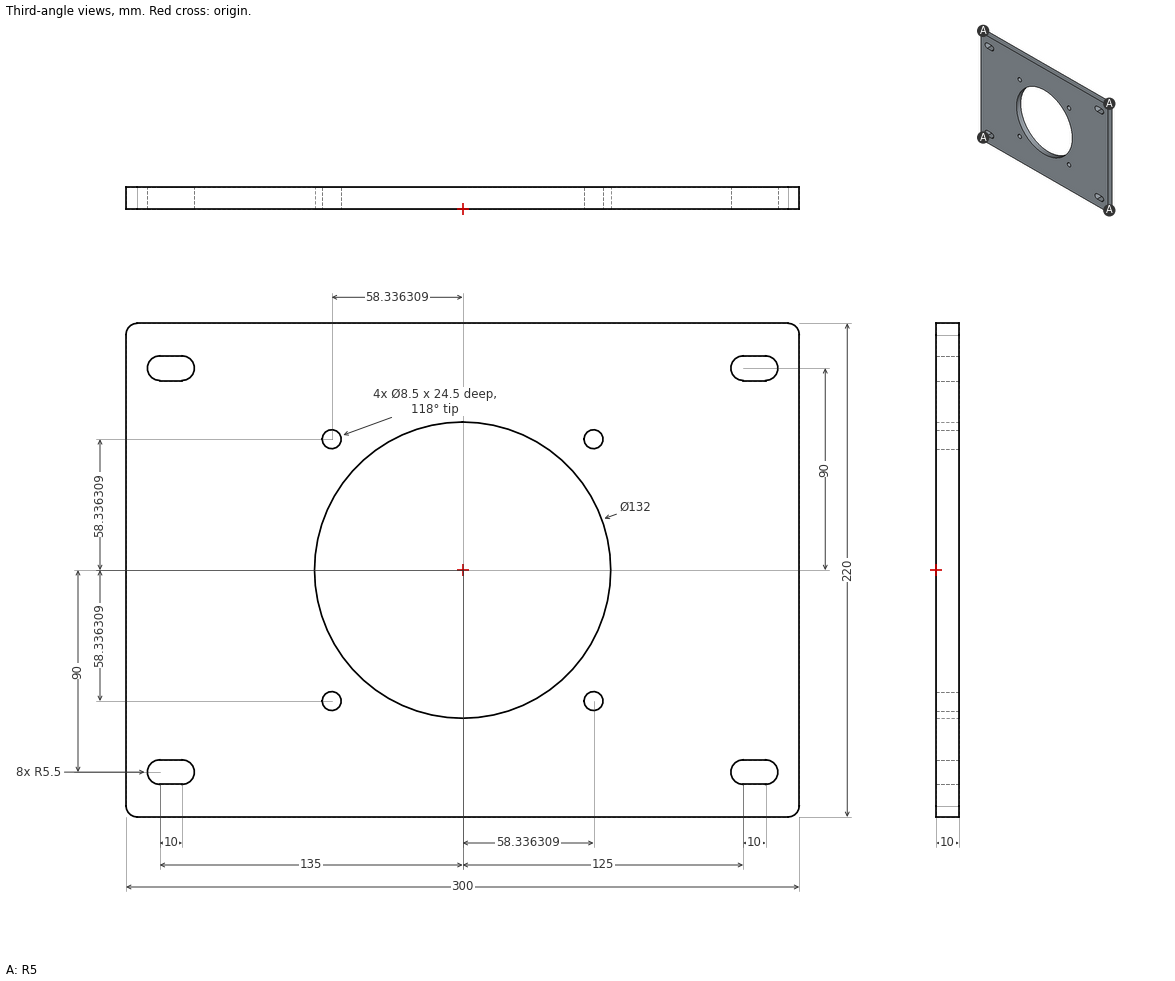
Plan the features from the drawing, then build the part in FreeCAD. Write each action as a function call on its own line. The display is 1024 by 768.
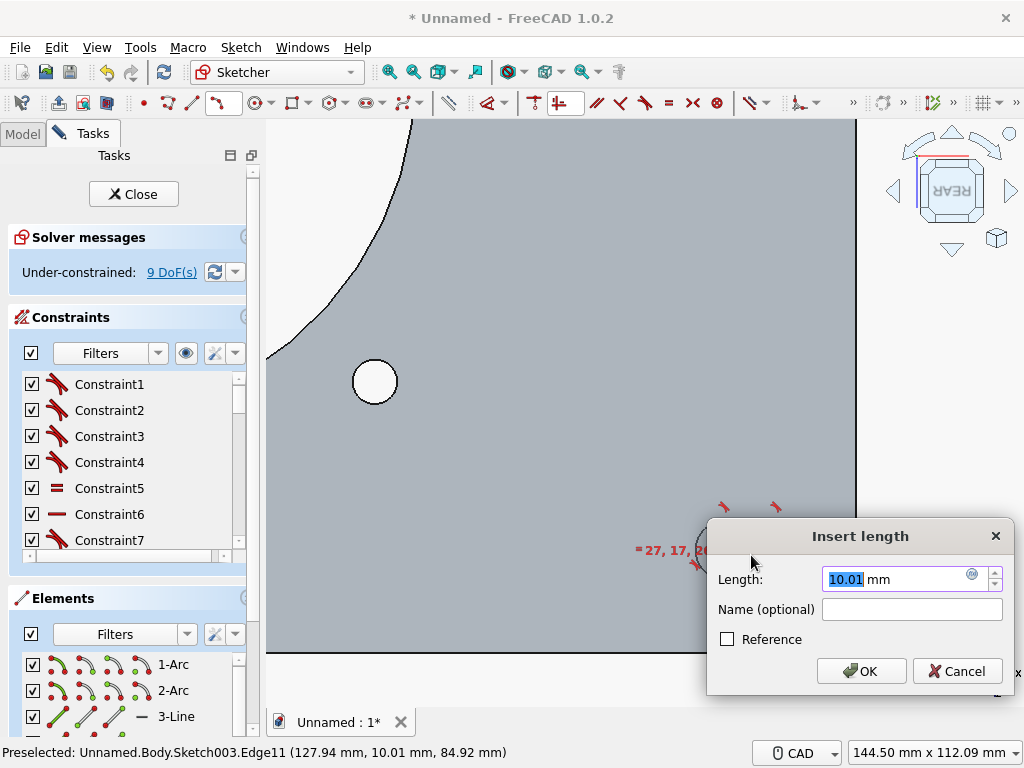
text(10)
key(Return)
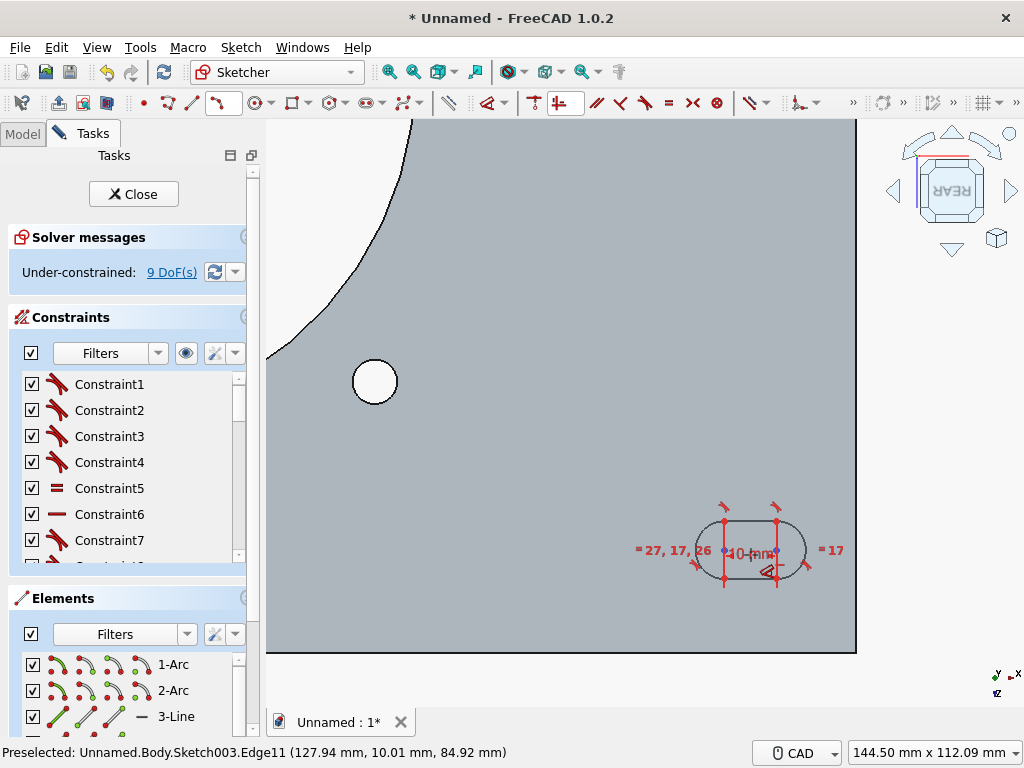
scroll(743, 523, down, 7)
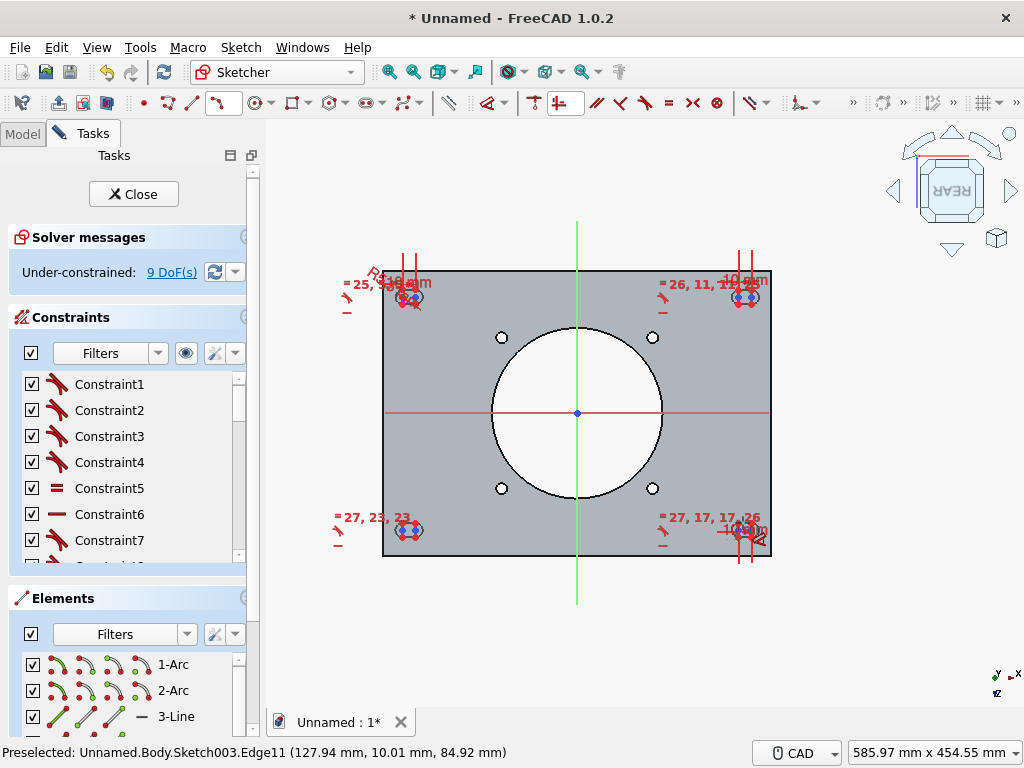
scroll(406, 523, up, 7)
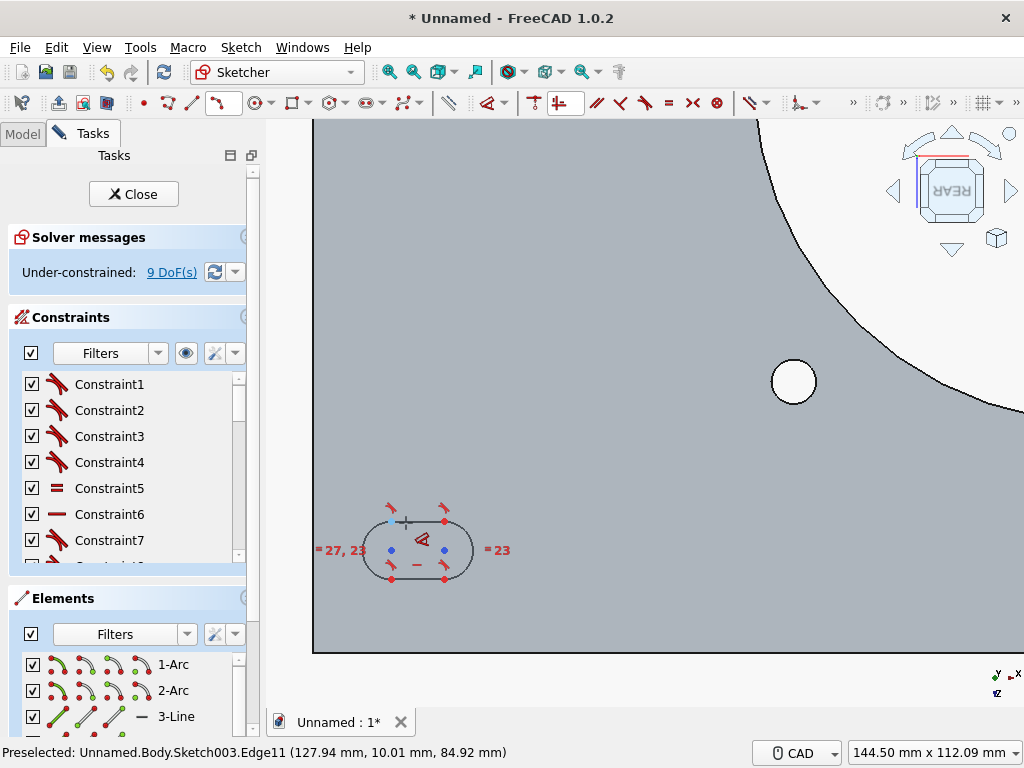
click(407, 522)
click(418, 556)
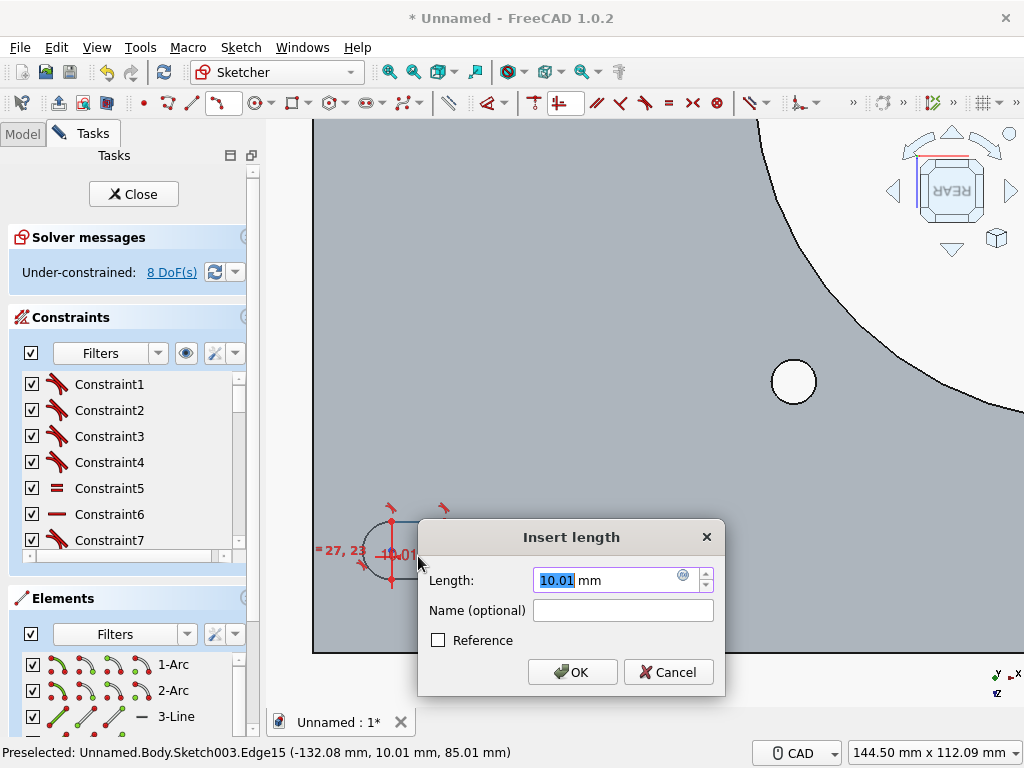
text(10)
key(Return)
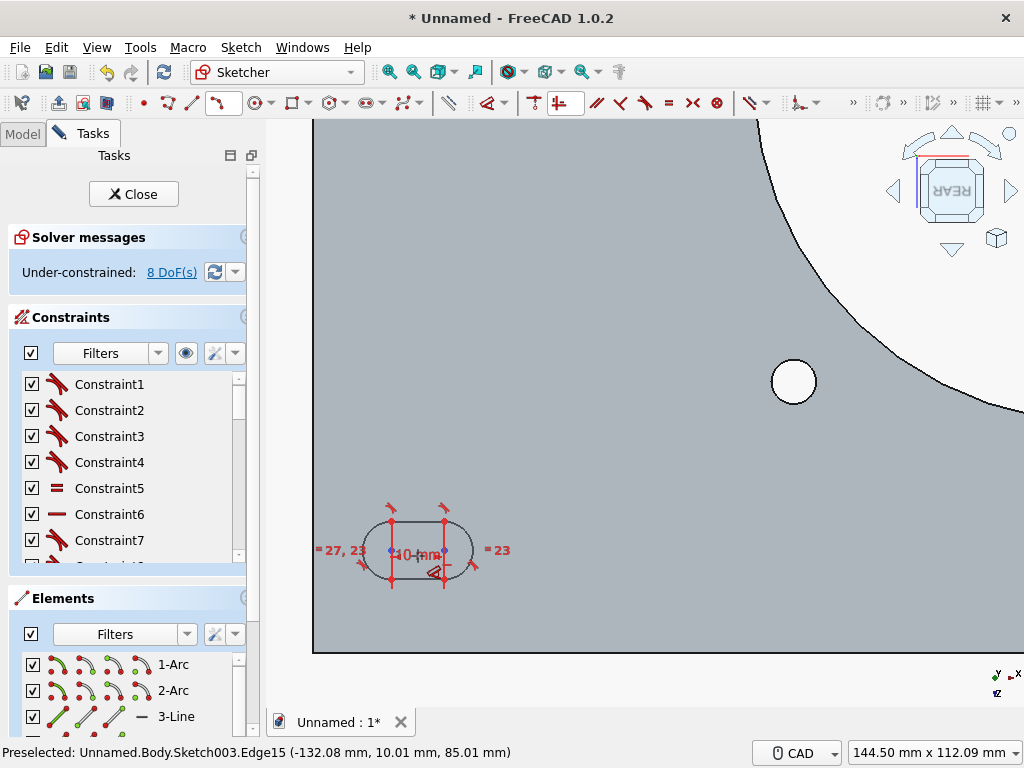
scroll(405, 523, down, 7)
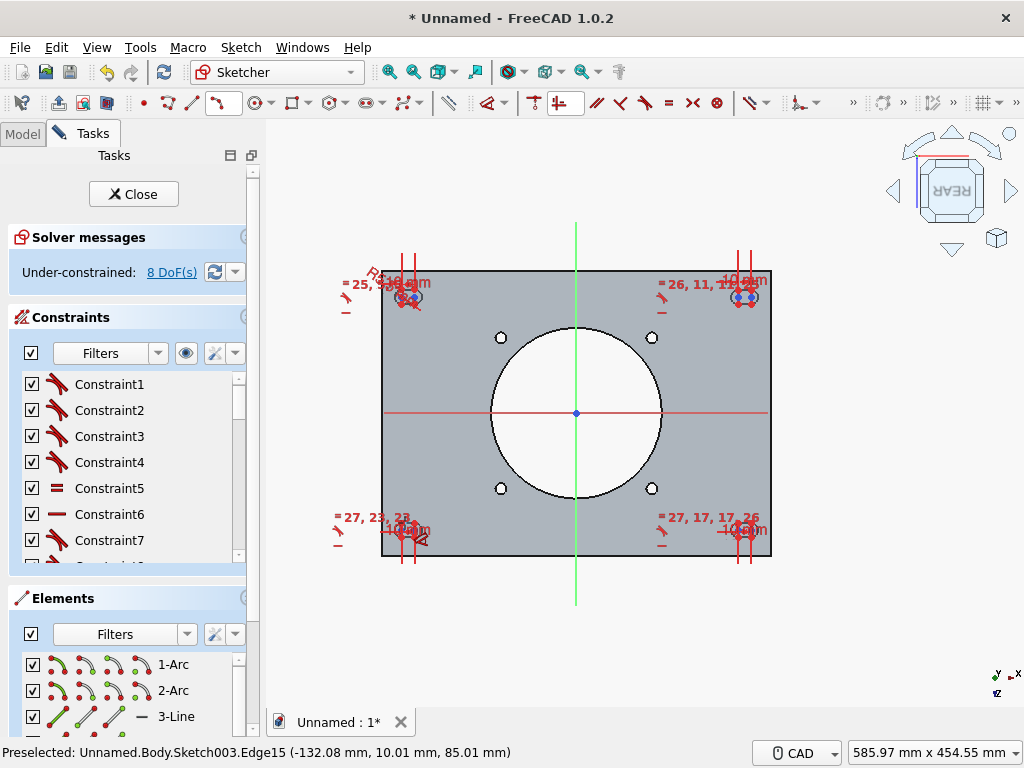
scroll(402, 297, up, 3)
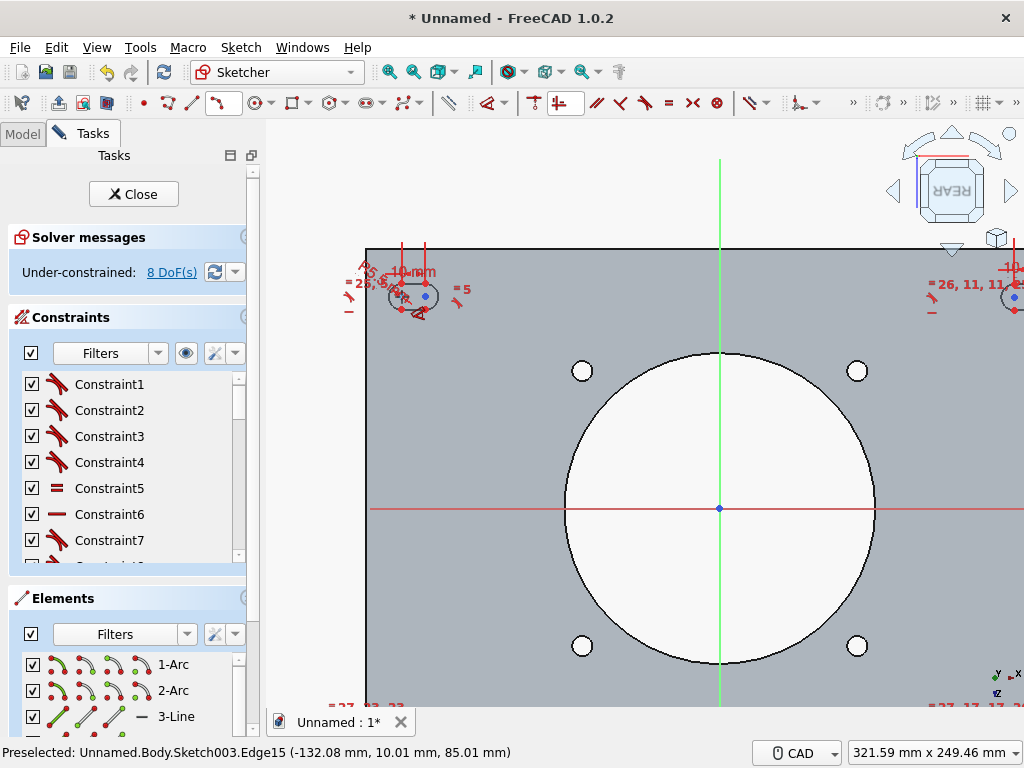
click(402, 297)
click(368, 403)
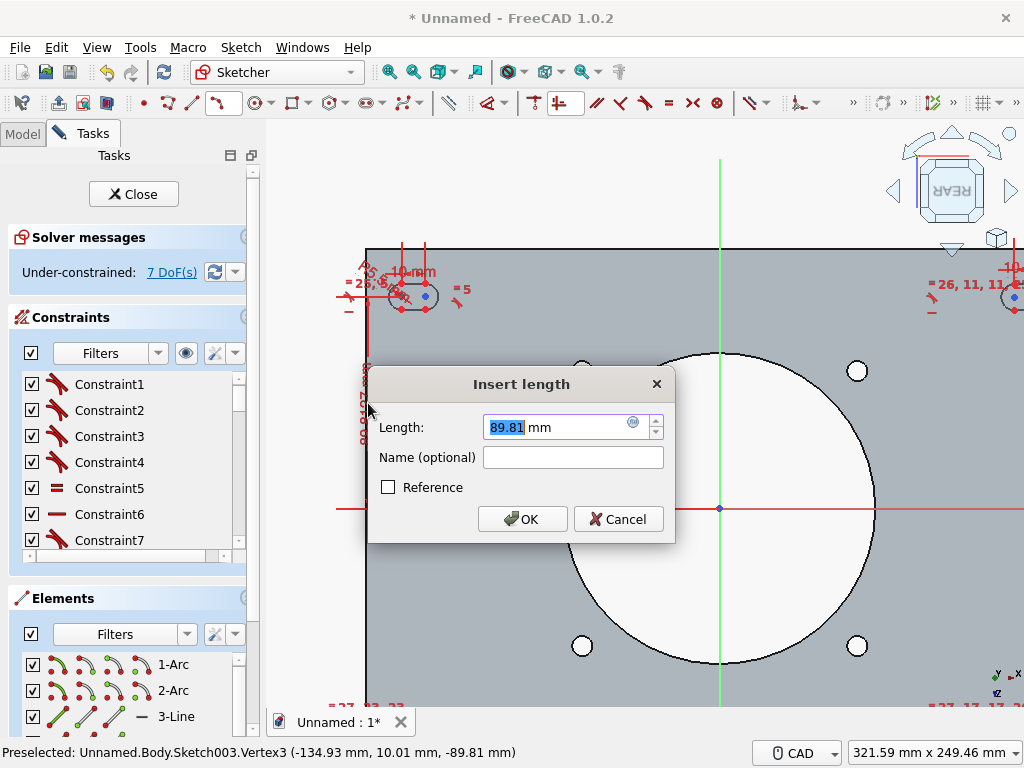
text(90)
key(Return)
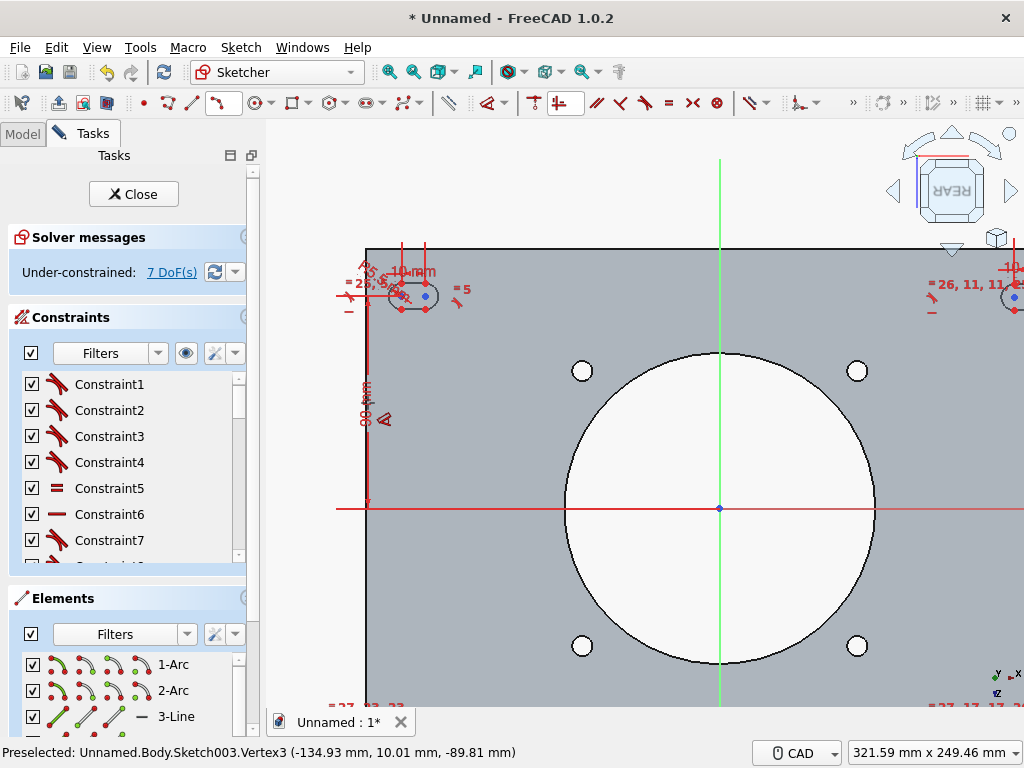
scroll(402, 297, down, 3)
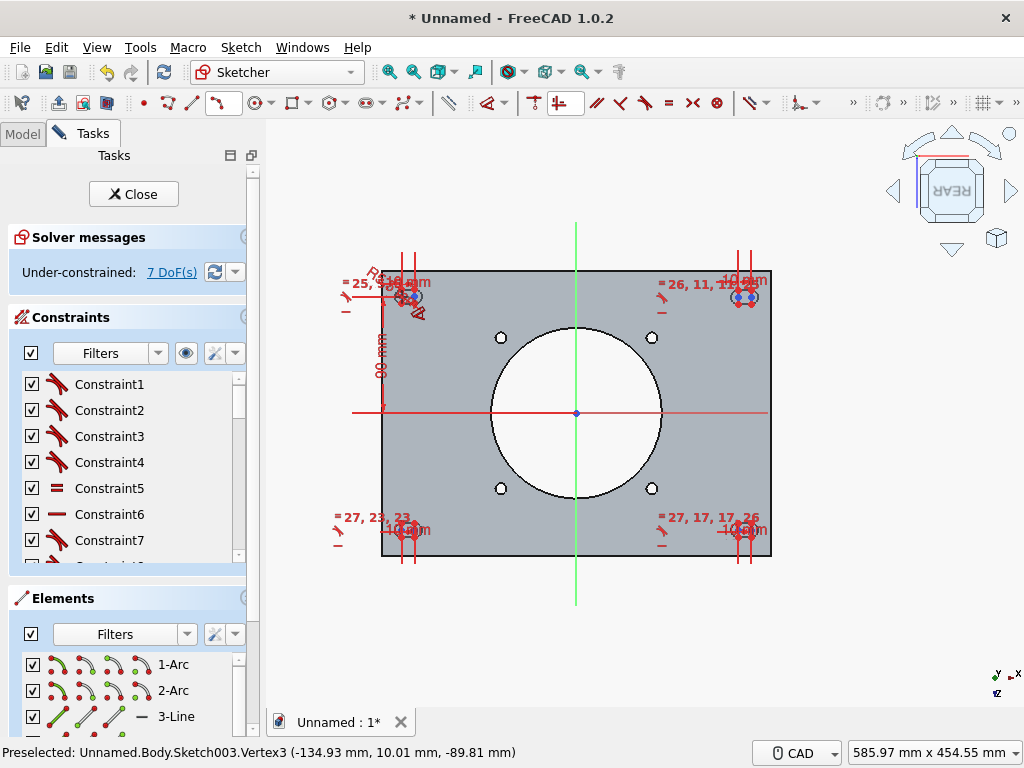
scroll(738, 297, up, 3)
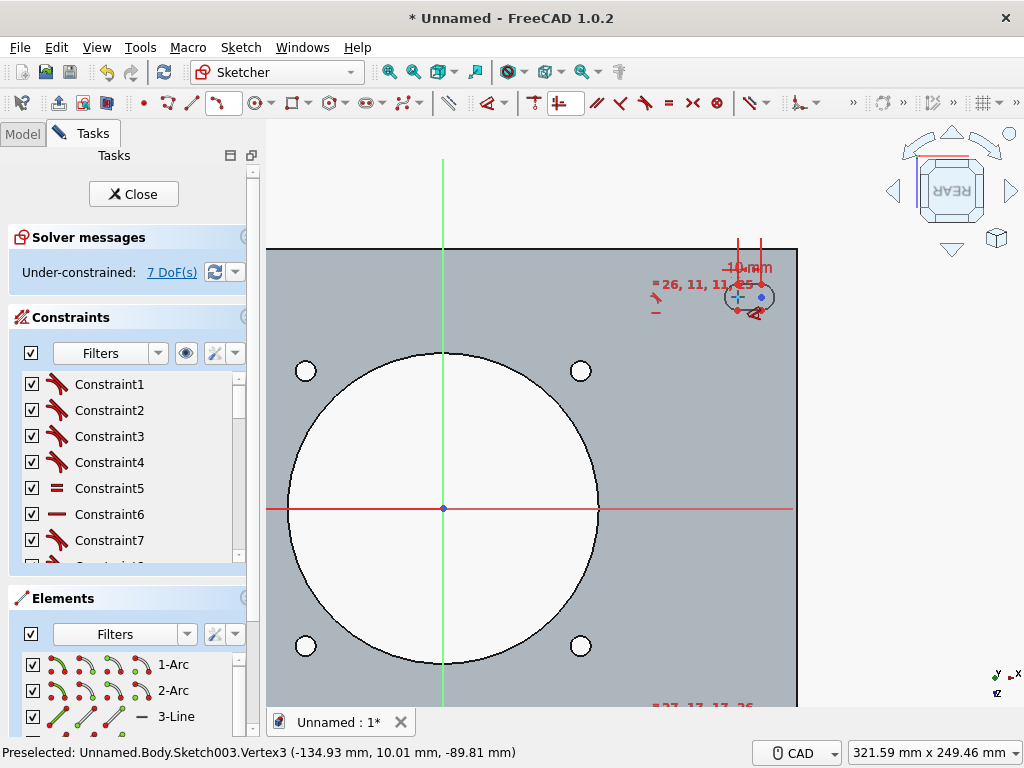
click(738, 297)
click(772, 403)